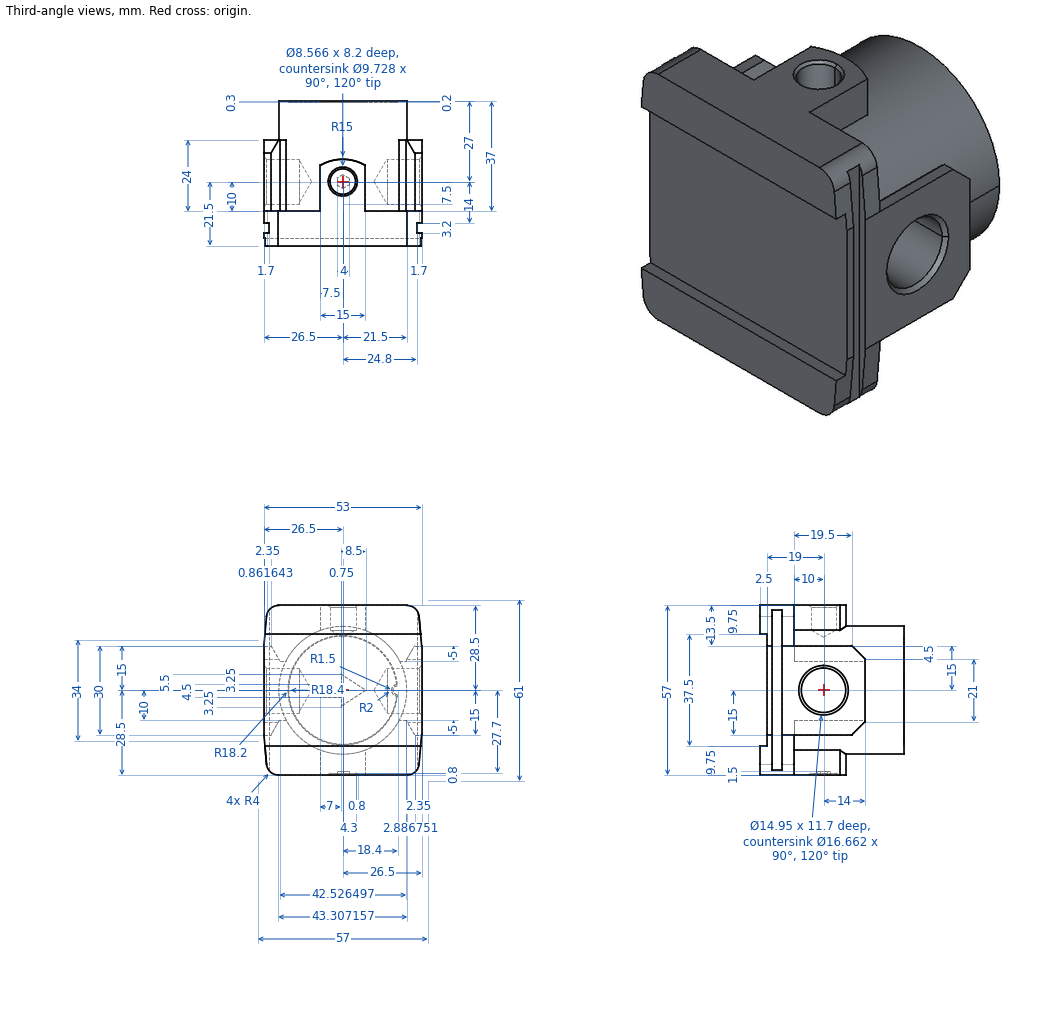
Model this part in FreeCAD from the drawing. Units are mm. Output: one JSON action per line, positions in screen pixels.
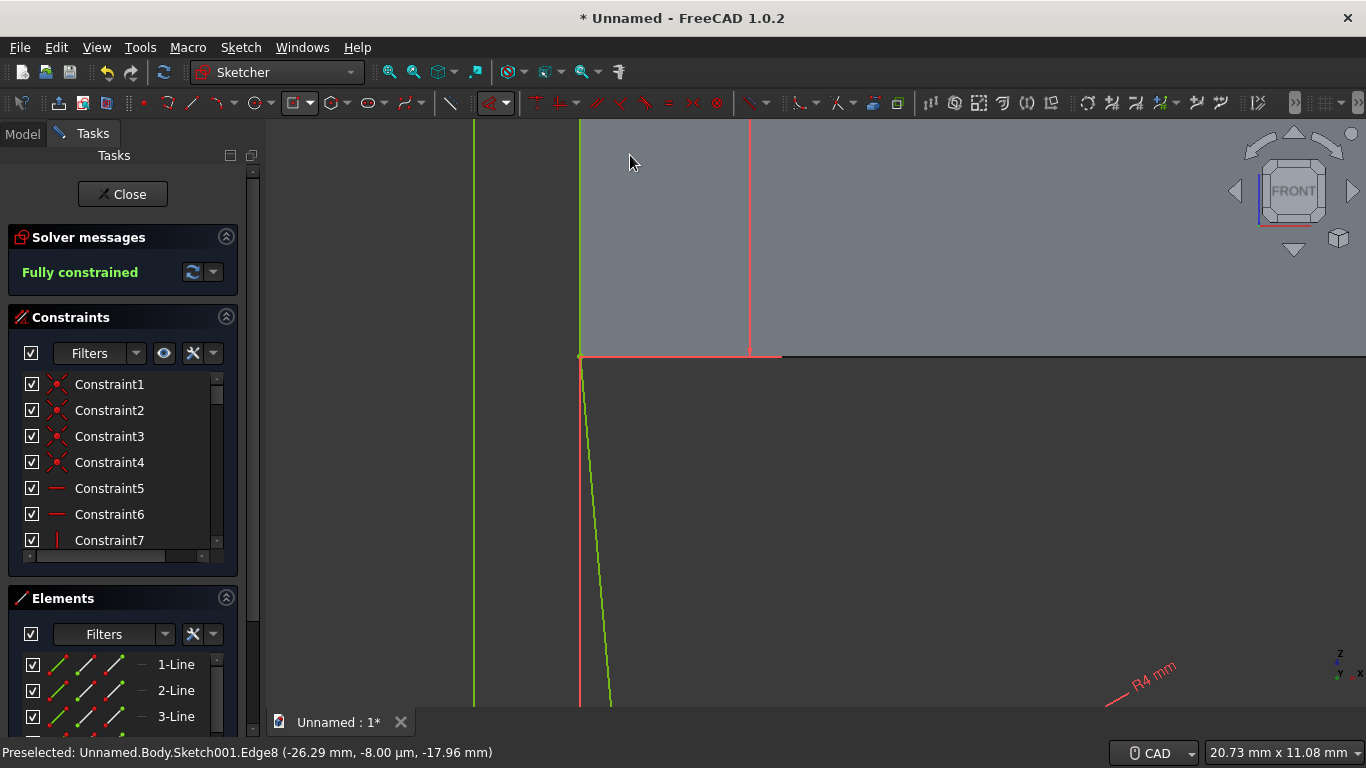
{"action": "left_click", "coordinate": [123, 194]}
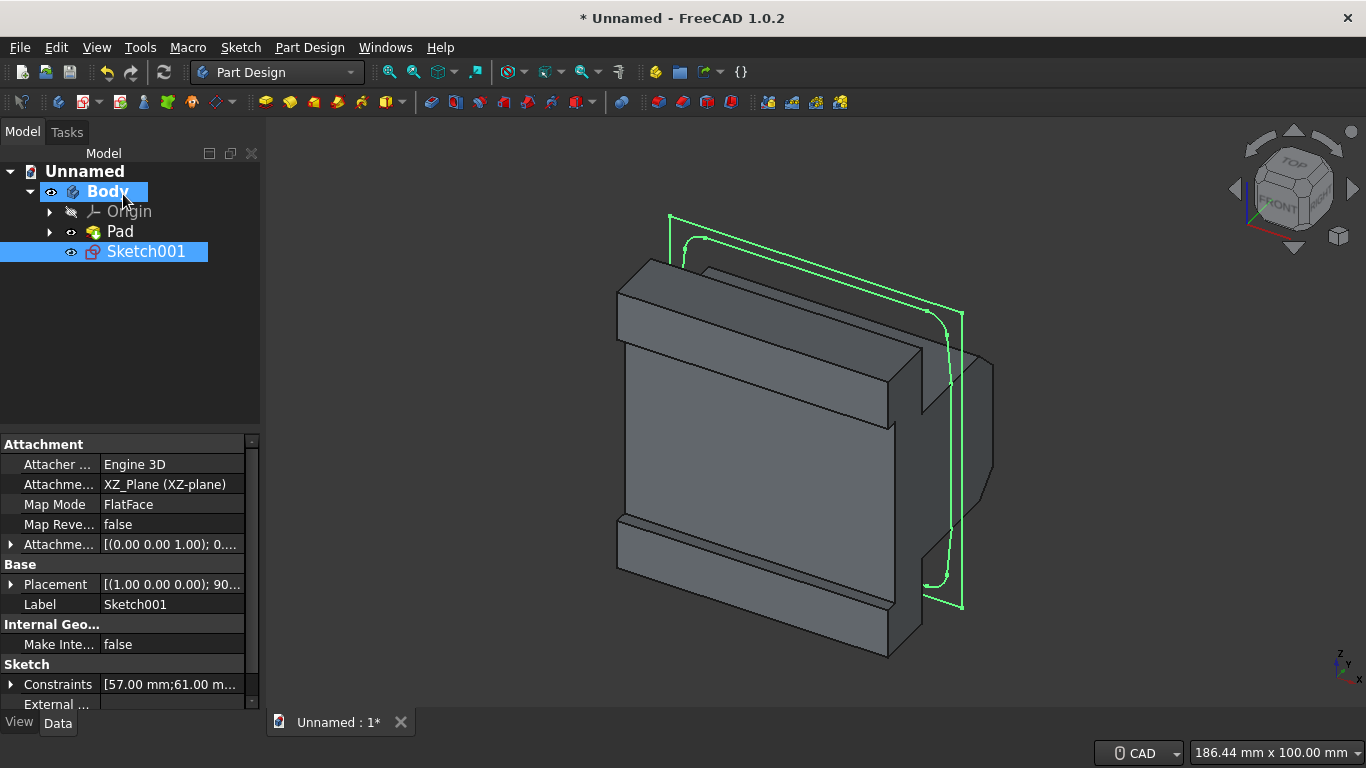
{"action": "left_click", "coordinate": [432, 102]}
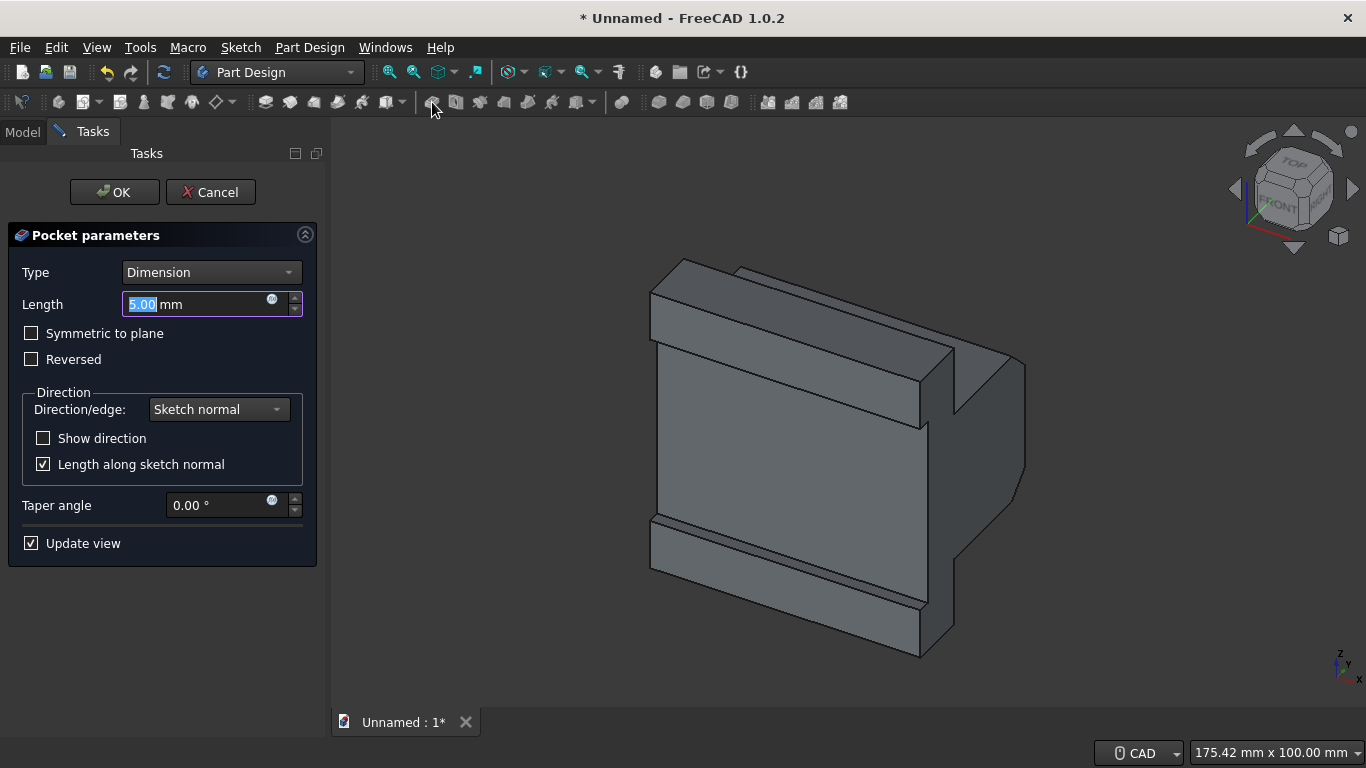
{"action": "type", "text": "21.5"}
{"action": "key", "text": "Tab"}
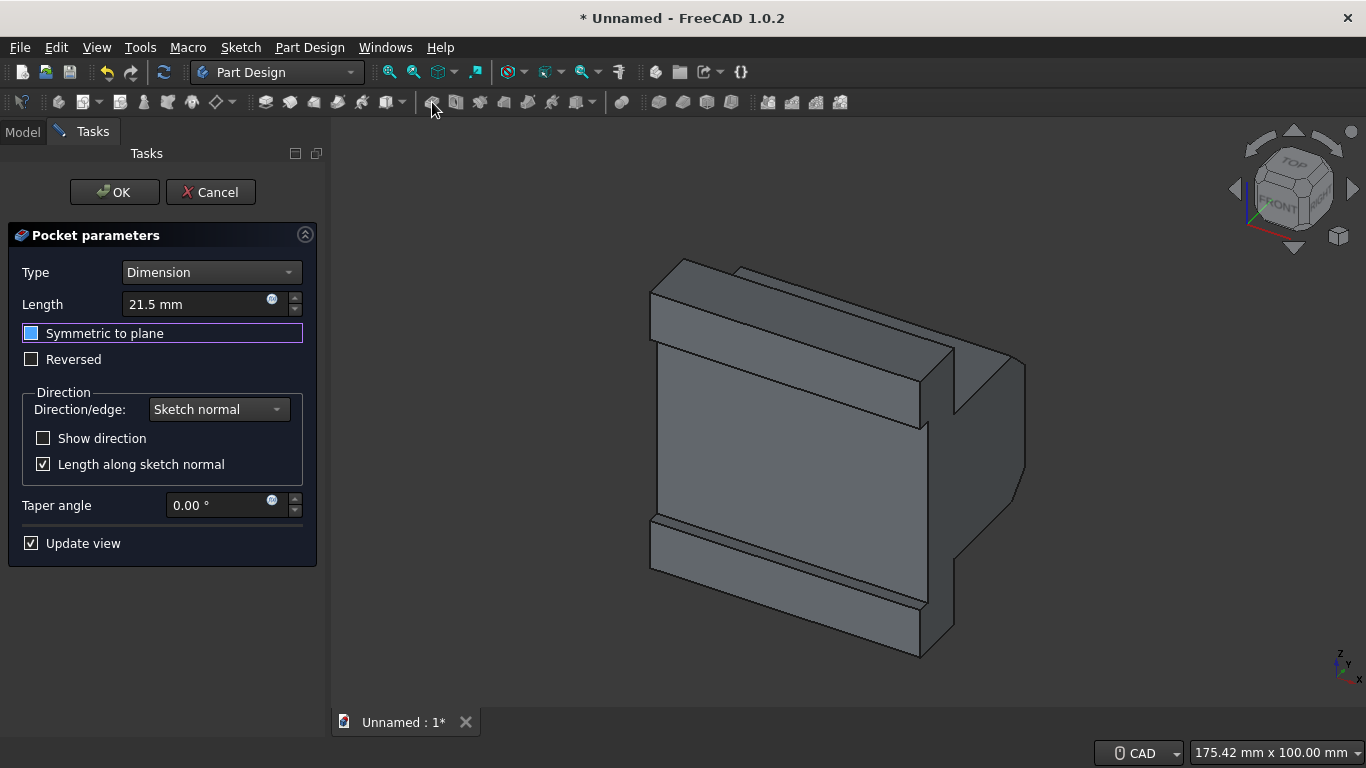
{"action": "left_click", "coordinate": [30, 359]}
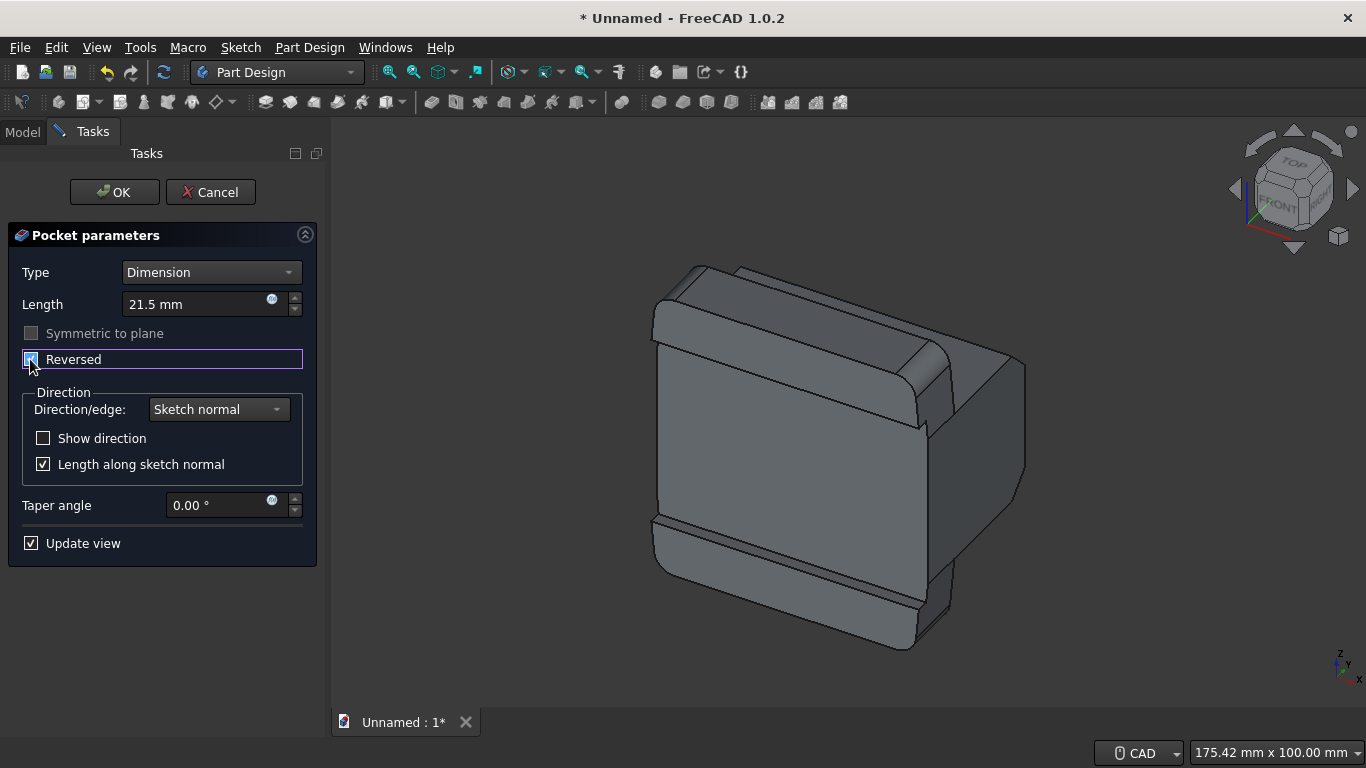
{"action": "left_click", "coordinate": [115, 192]}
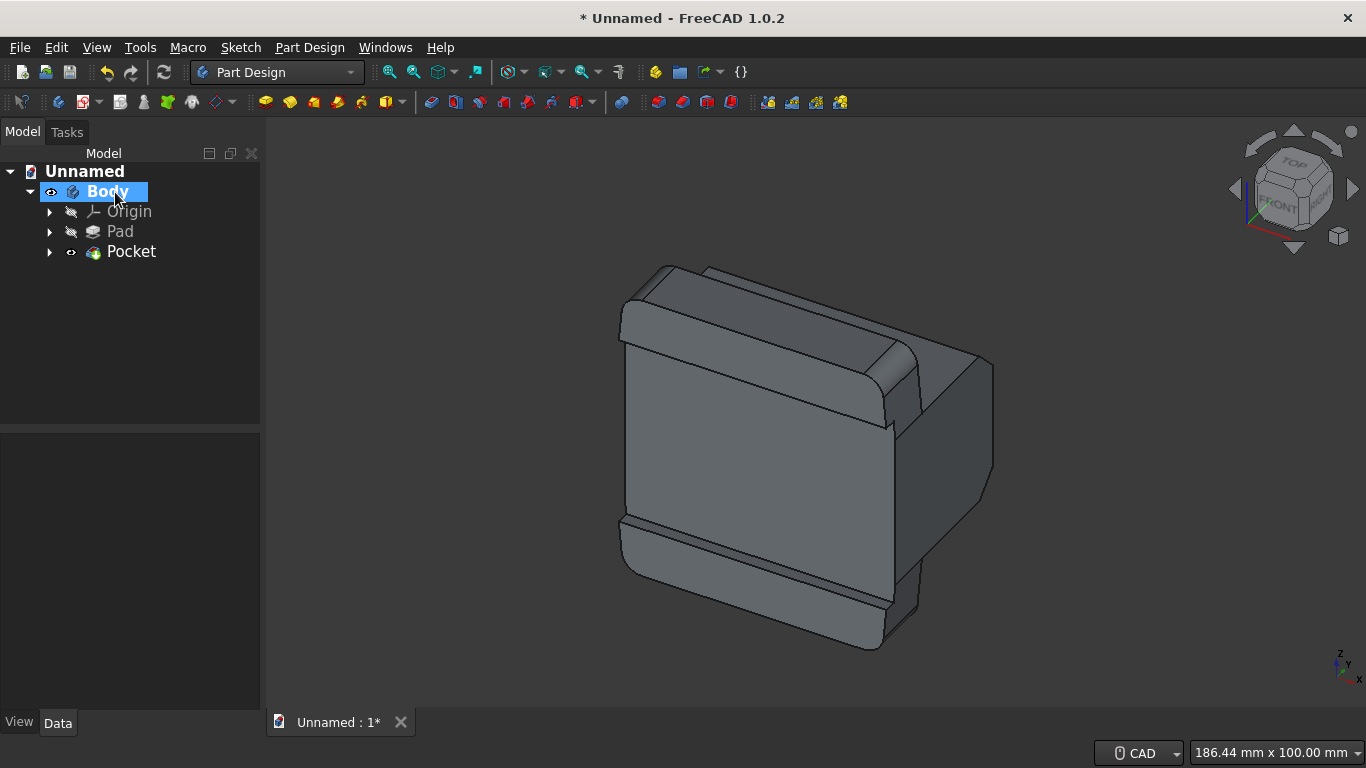
{"action": "key", "text": "4"}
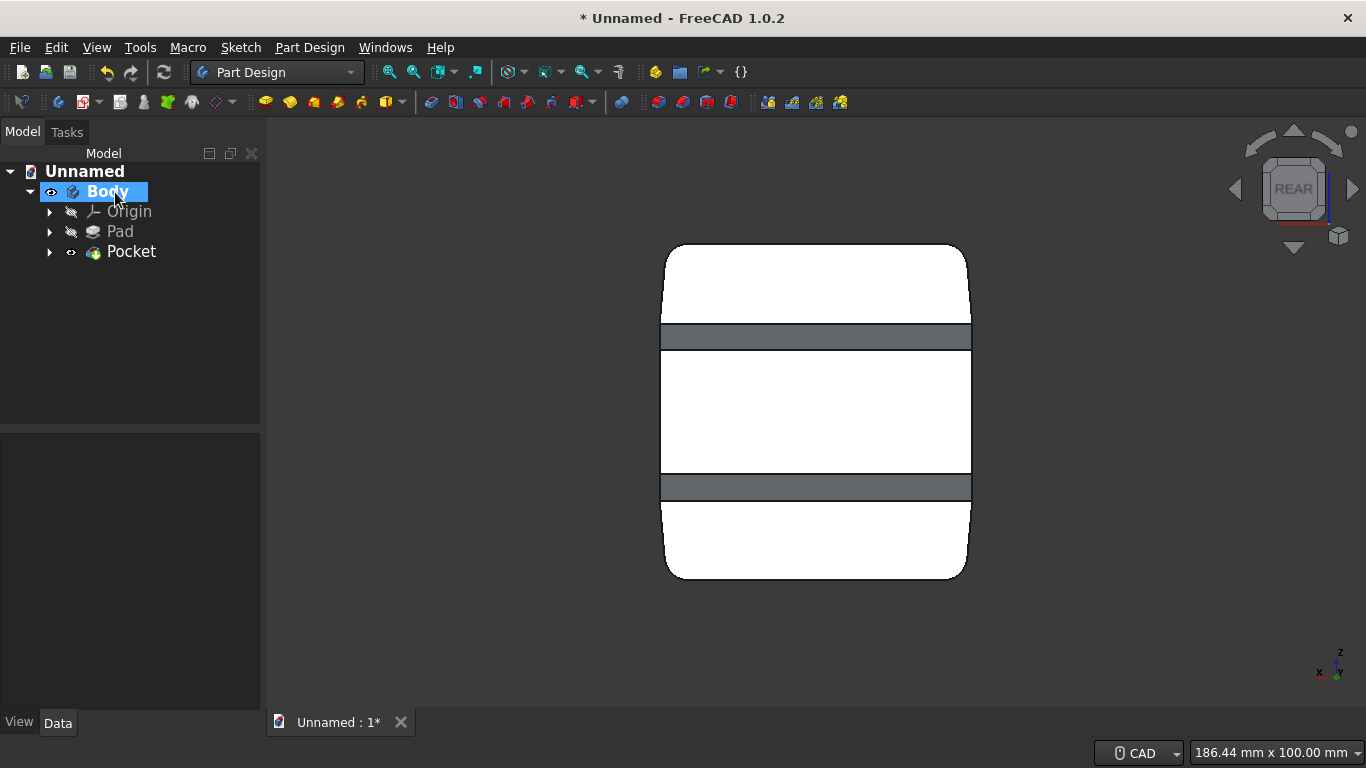
{"action": "left_click", "coordinate": [727, 283]}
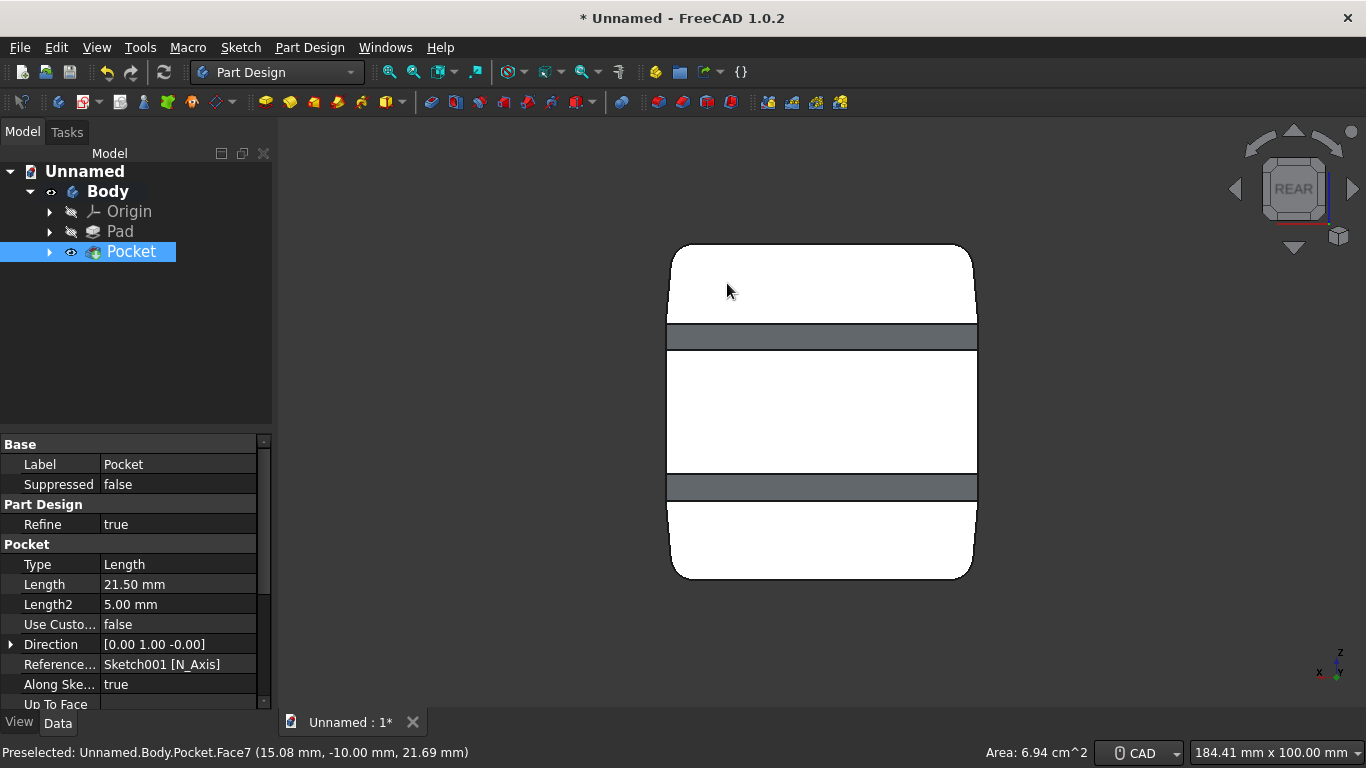
{"action": "left_click", "coordinate": [84, 102]}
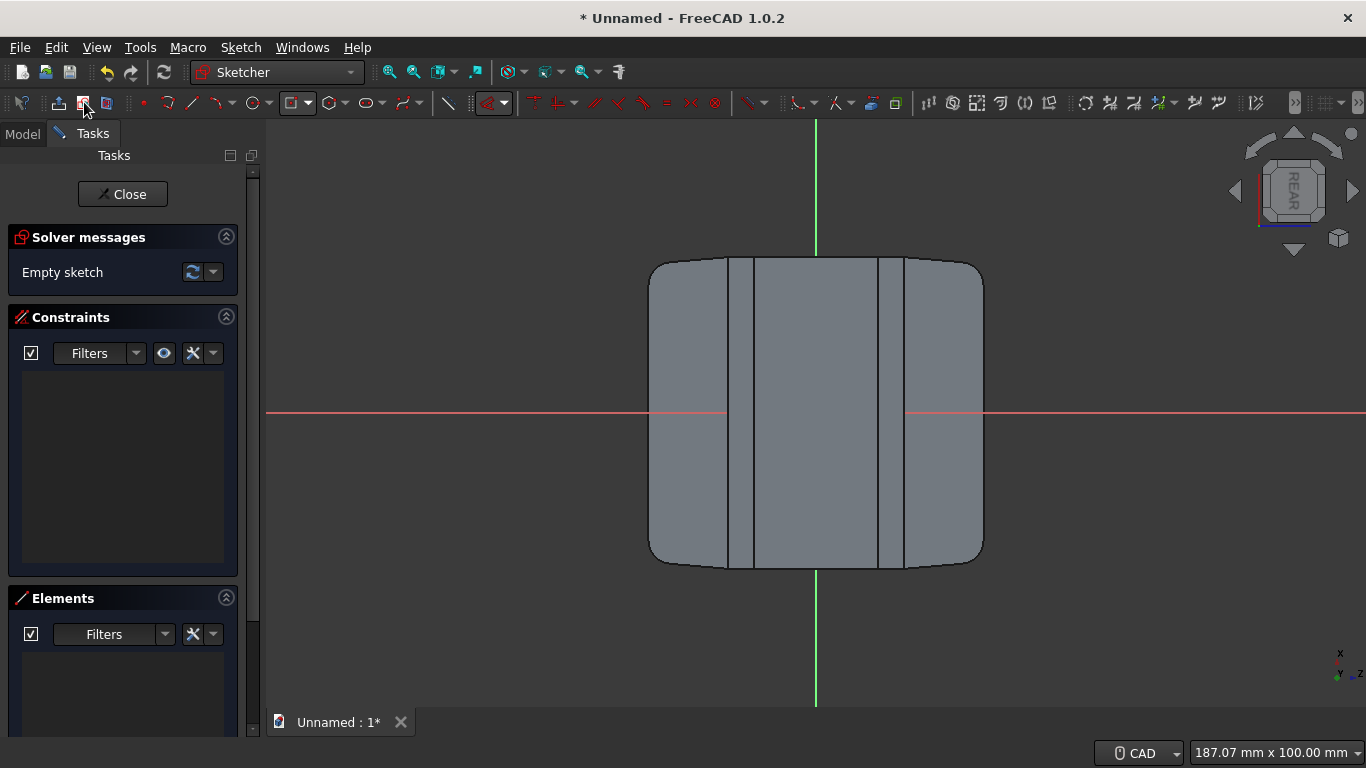
{"action": "left_click", "coordinate": [292, 104]}